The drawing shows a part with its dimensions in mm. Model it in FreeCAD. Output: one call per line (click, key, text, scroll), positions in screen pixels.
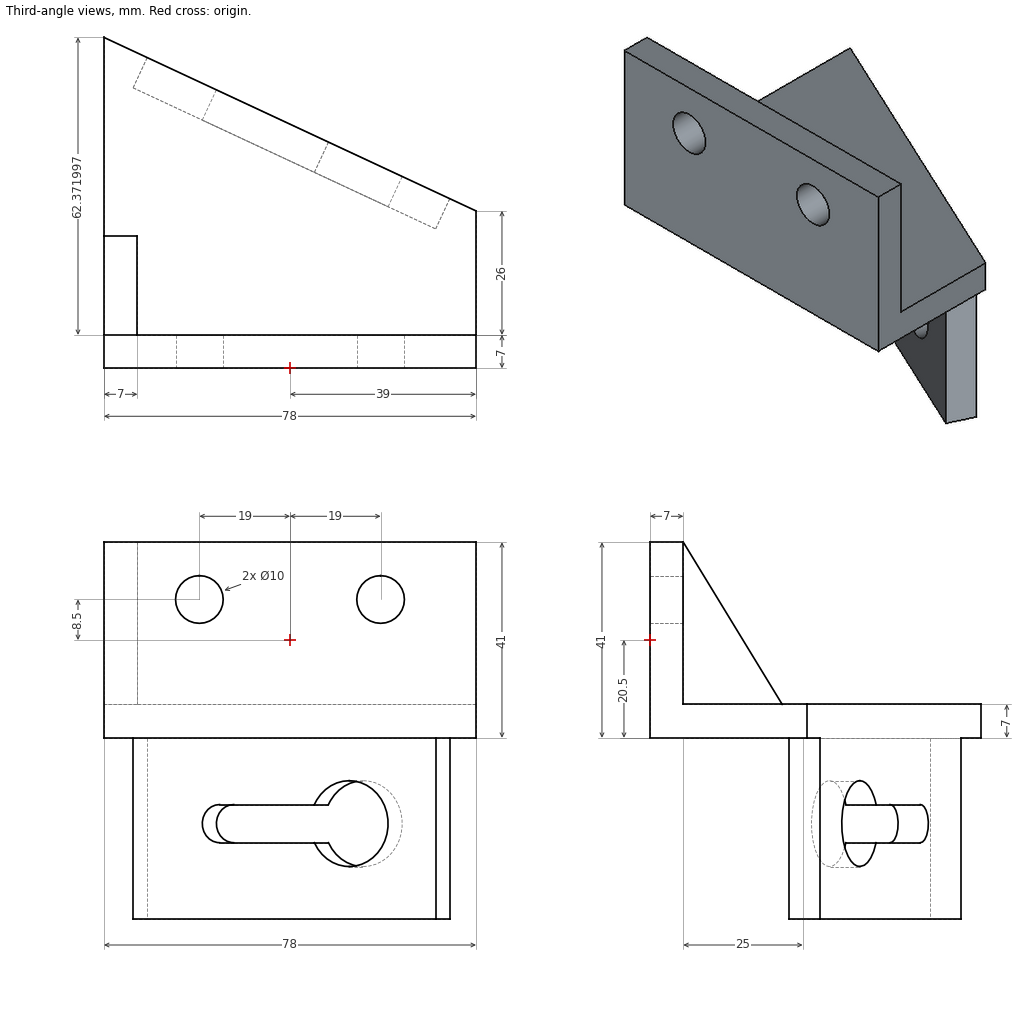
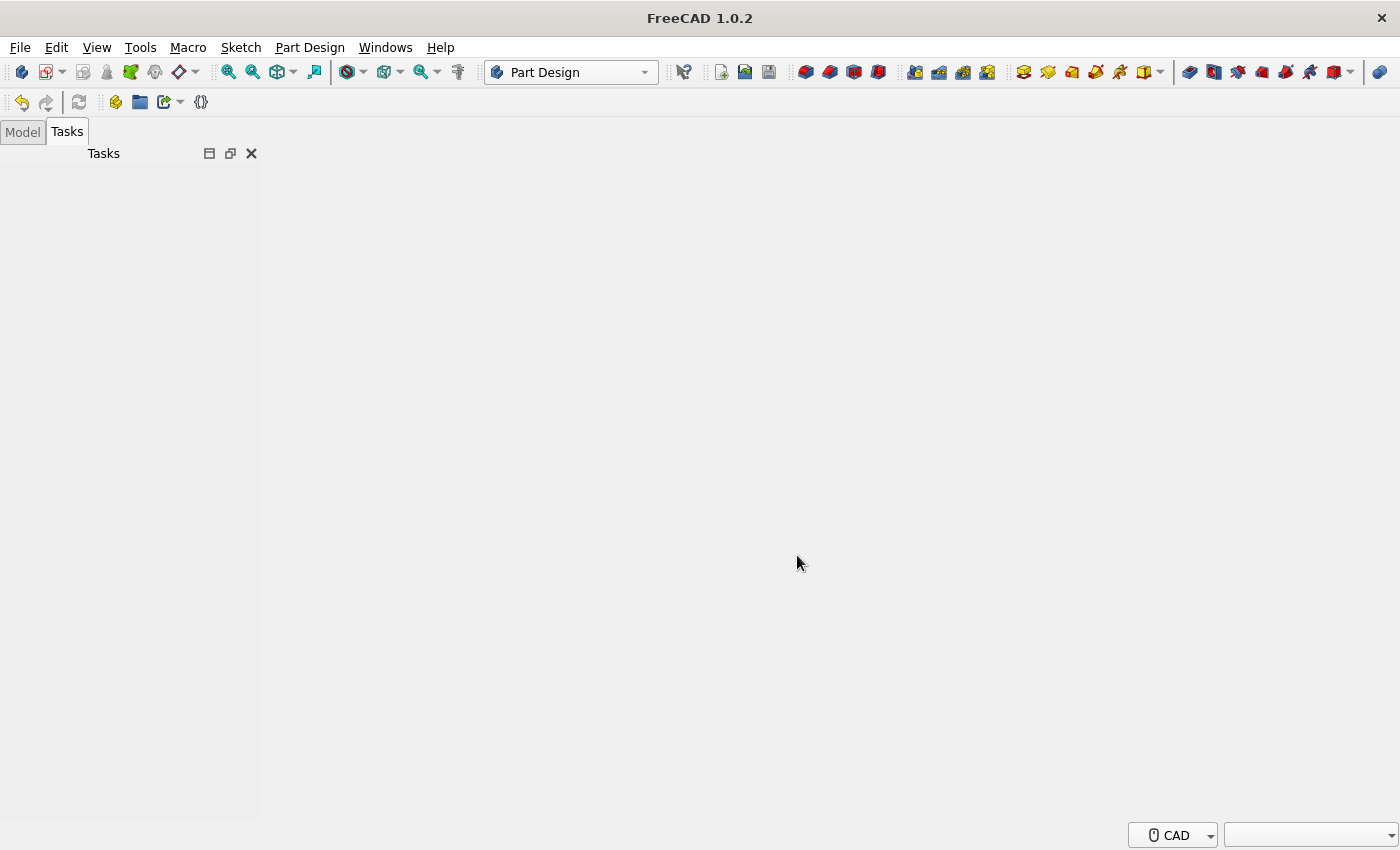
click(722, 72)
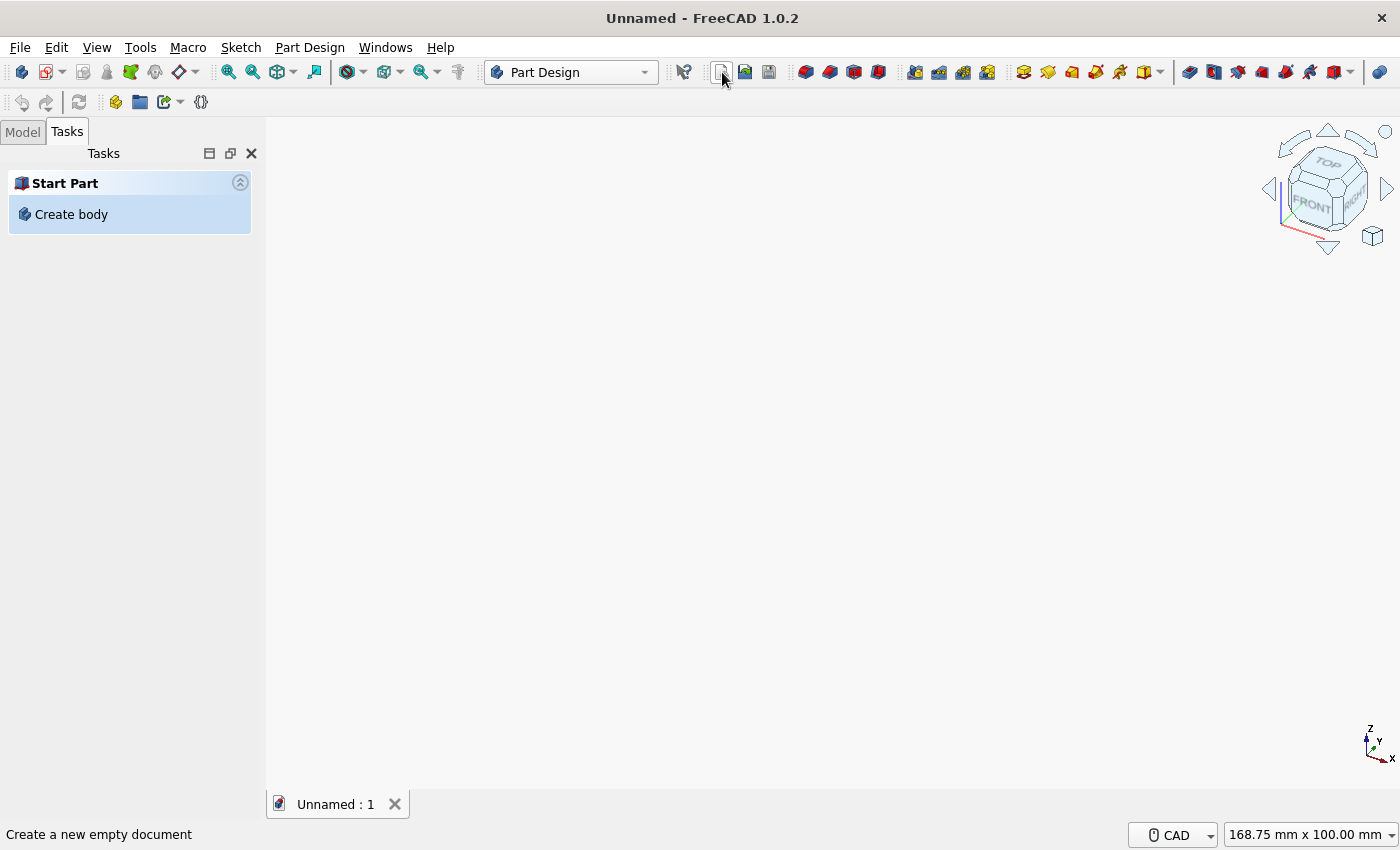
click(46, 72)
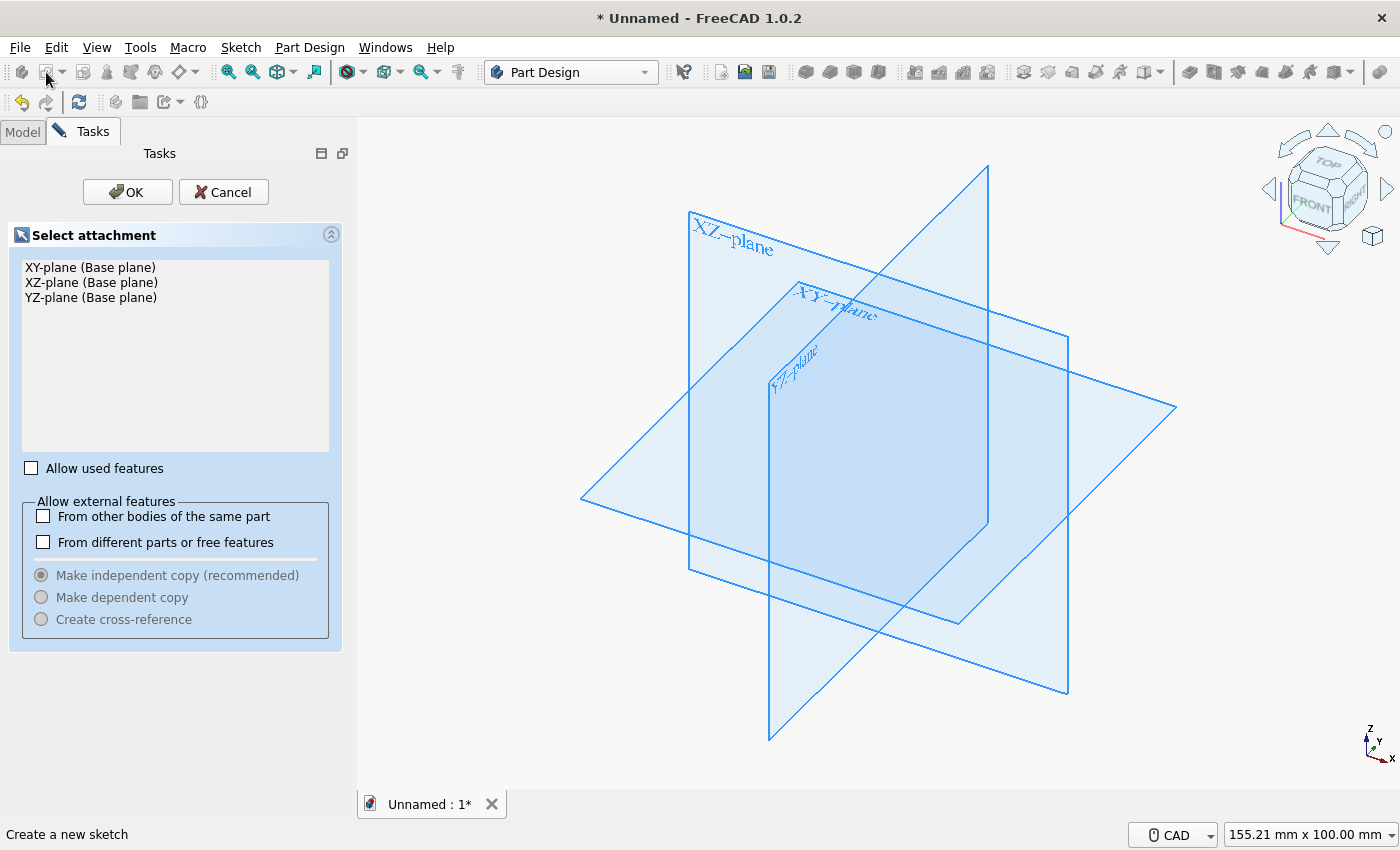
click(82, 282)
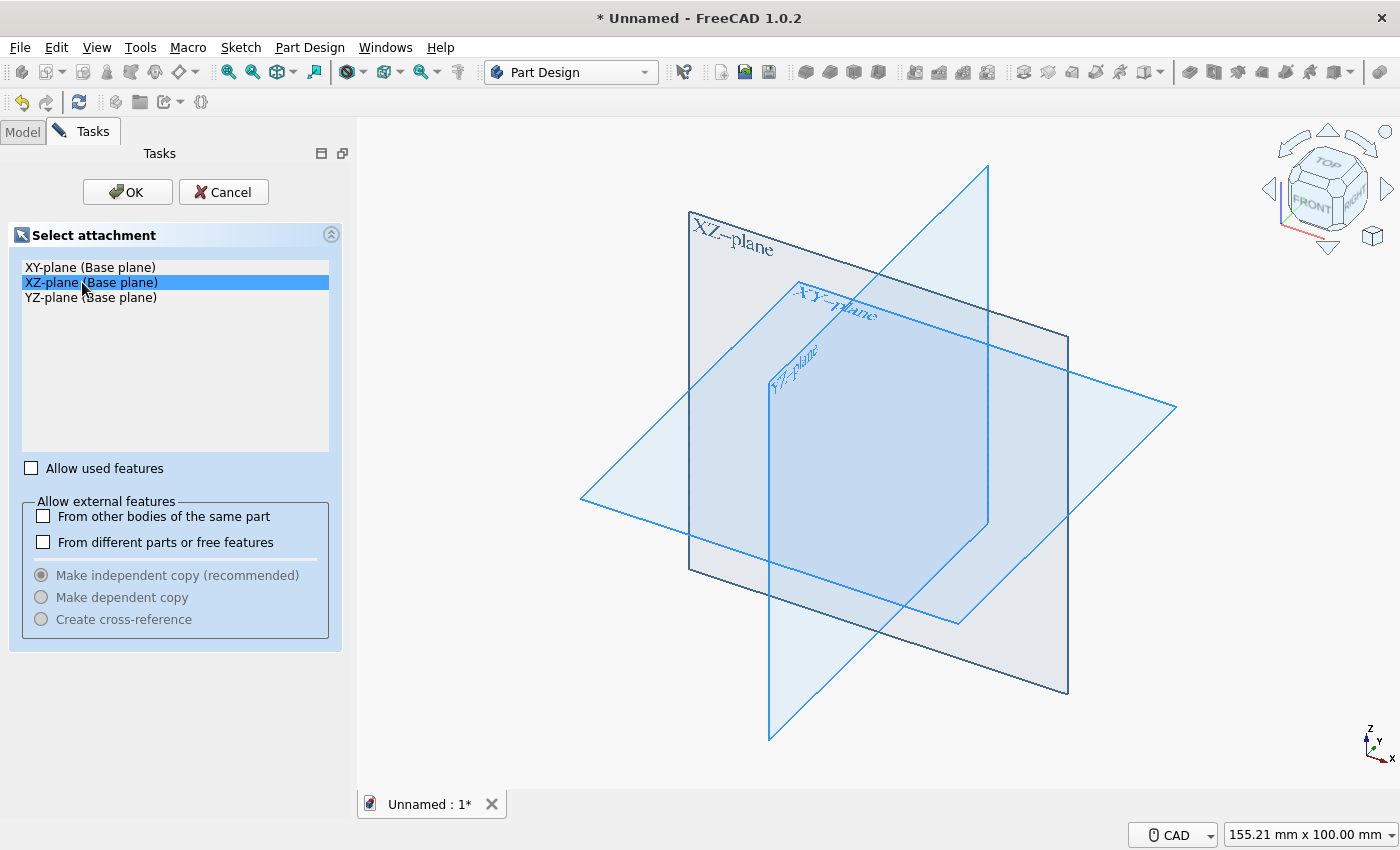
click(128, 192)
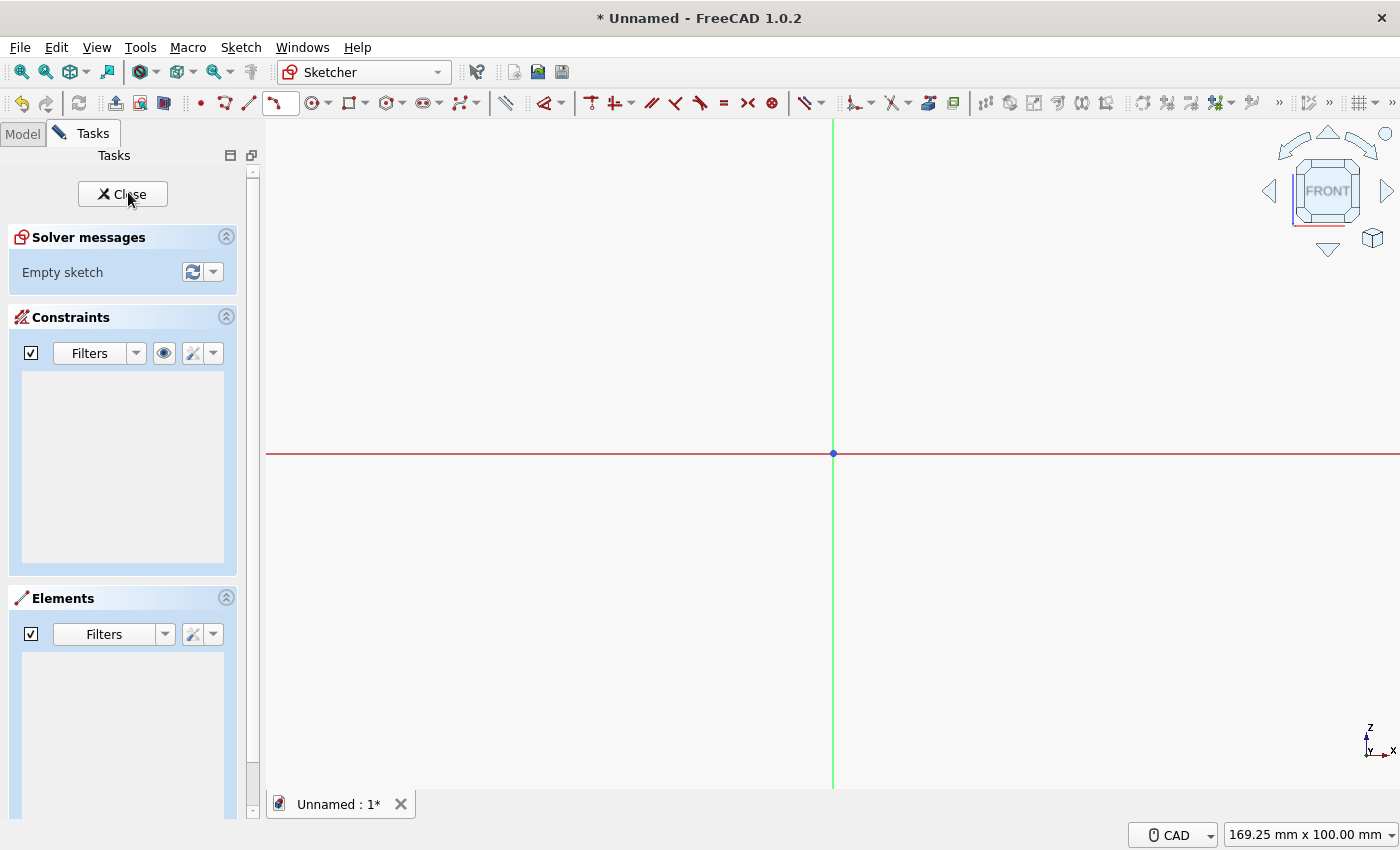
click(368, 104)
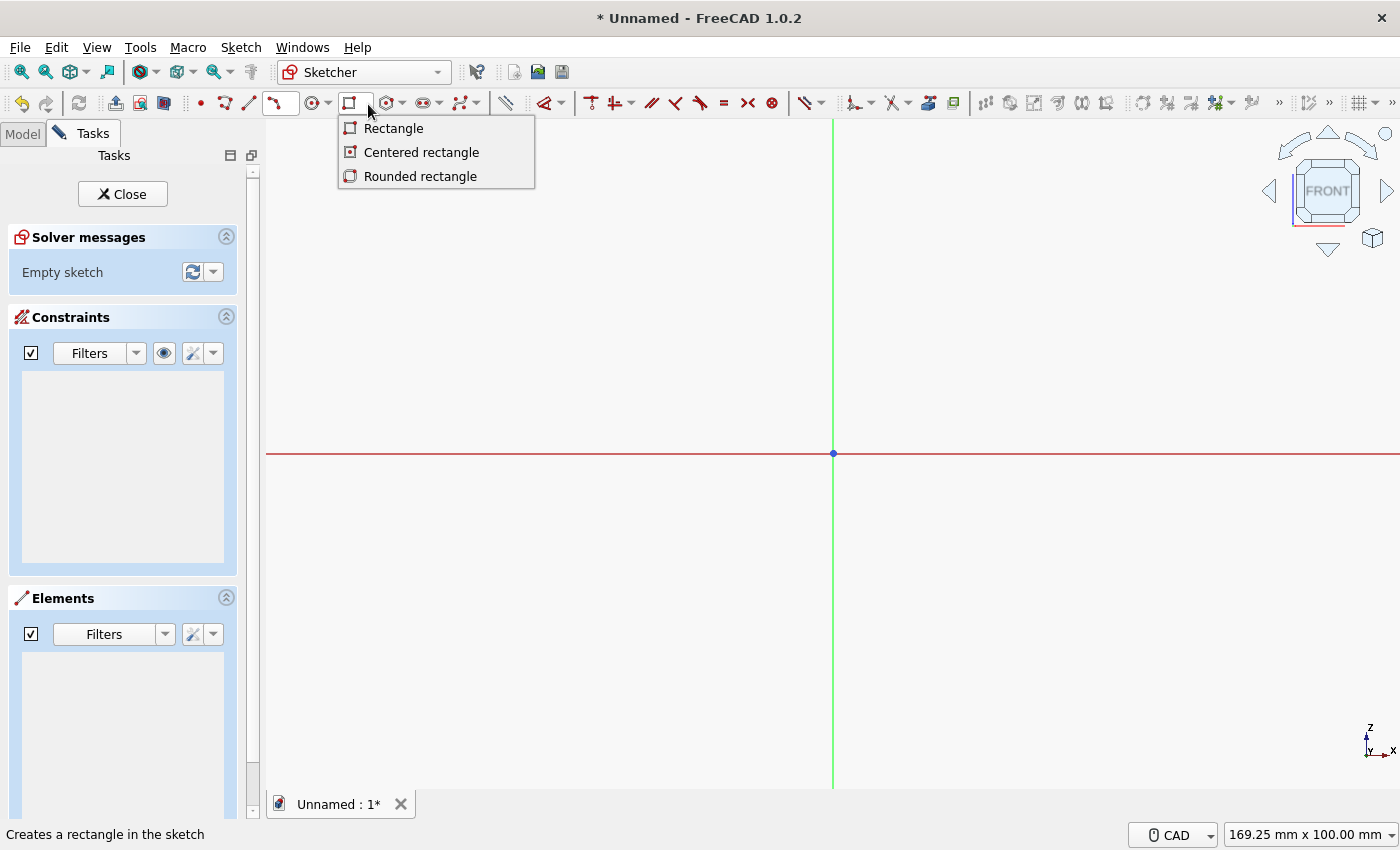
click(436, 152)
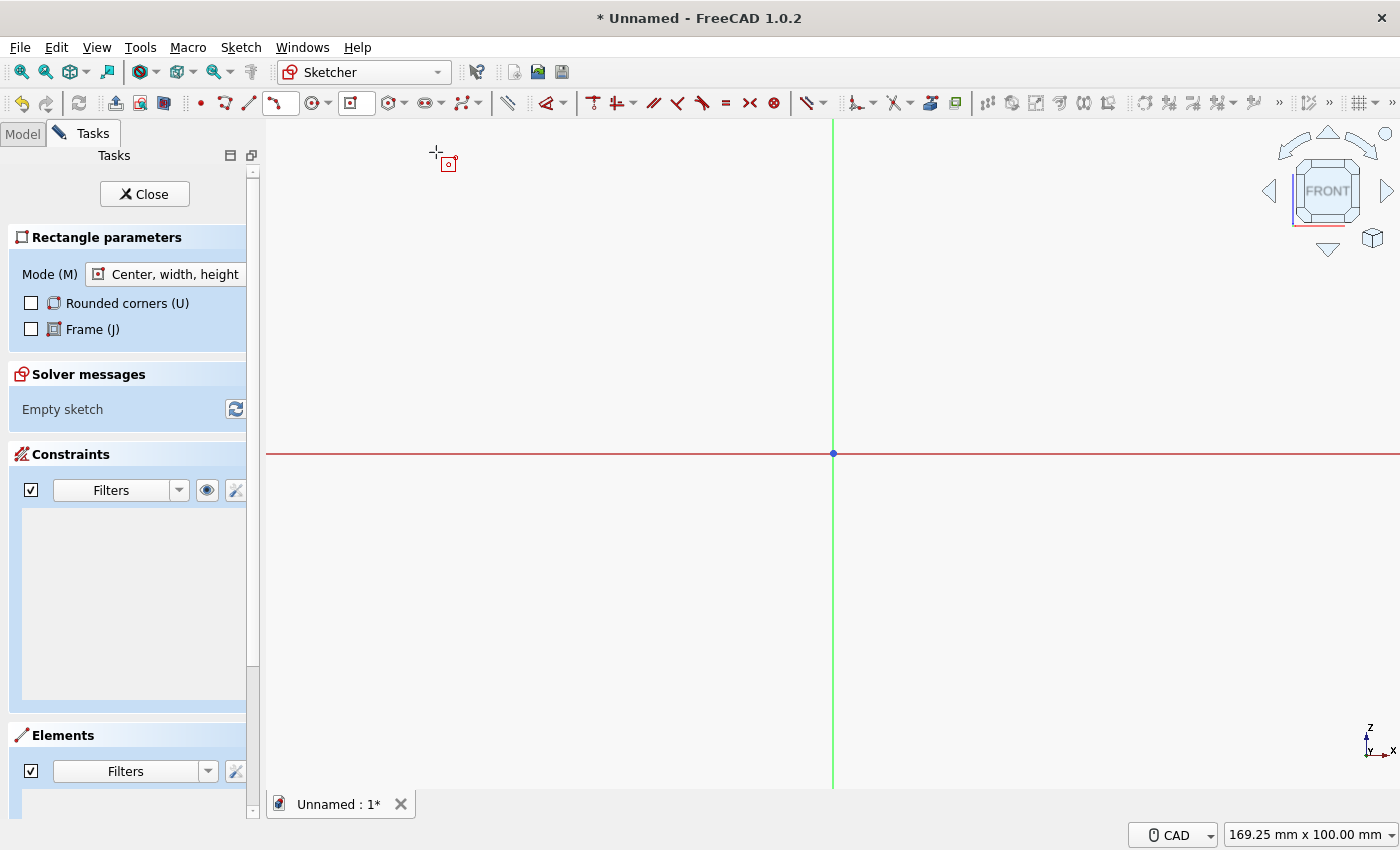
click(833, 454)
move(1094, 317)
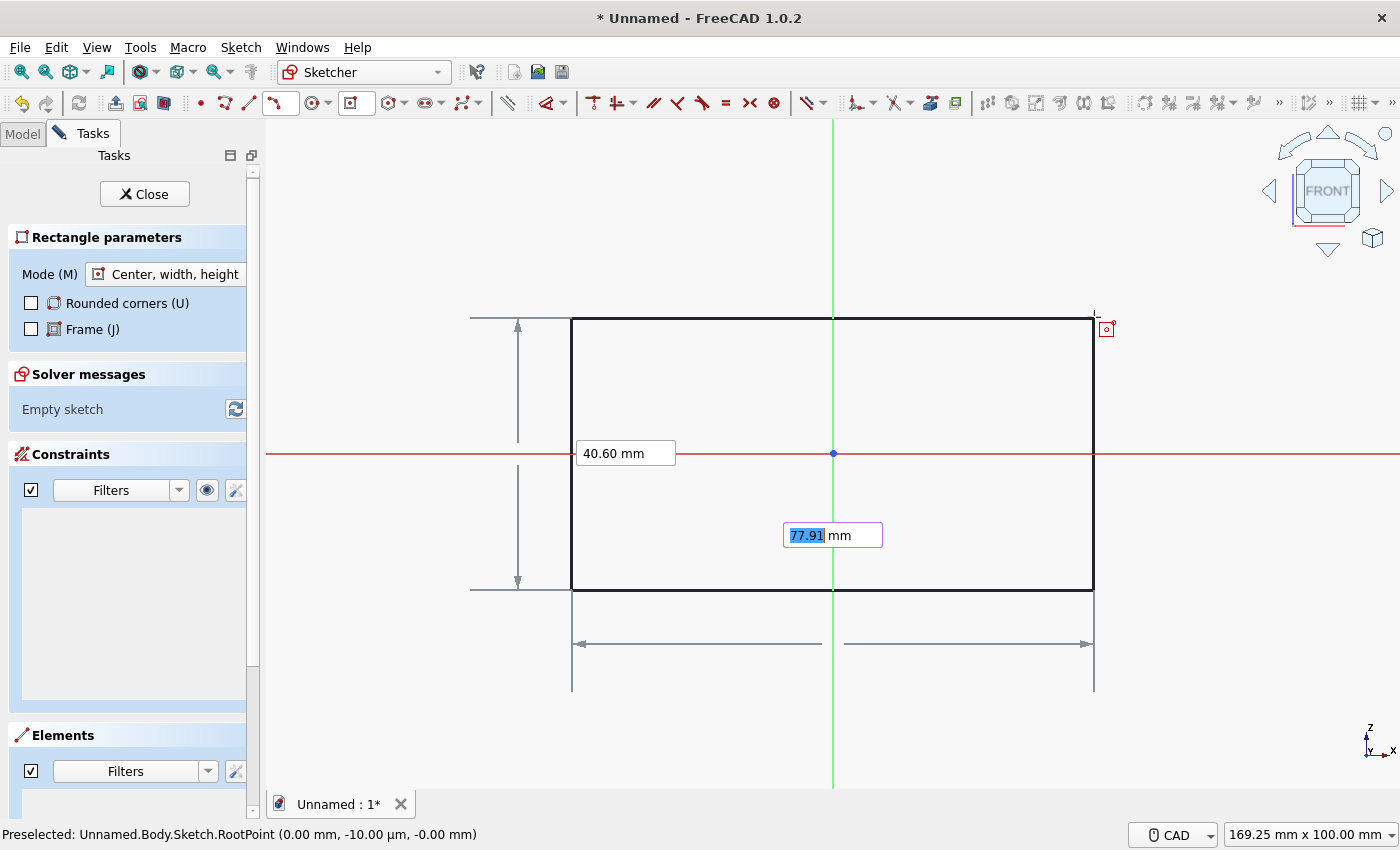
text(78)
key(Tab)
text(41)
key(Return)